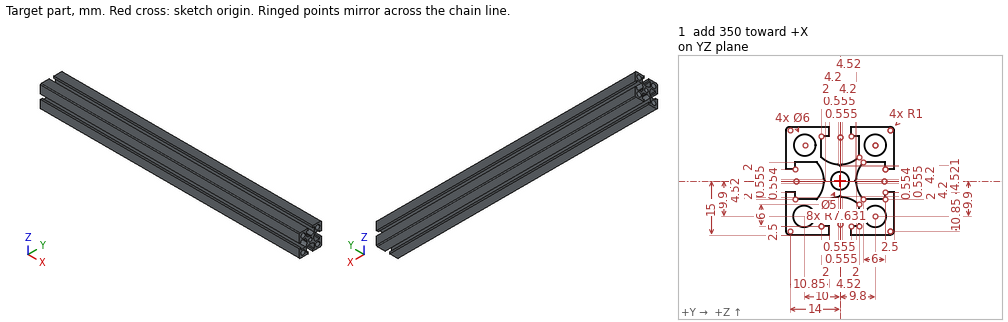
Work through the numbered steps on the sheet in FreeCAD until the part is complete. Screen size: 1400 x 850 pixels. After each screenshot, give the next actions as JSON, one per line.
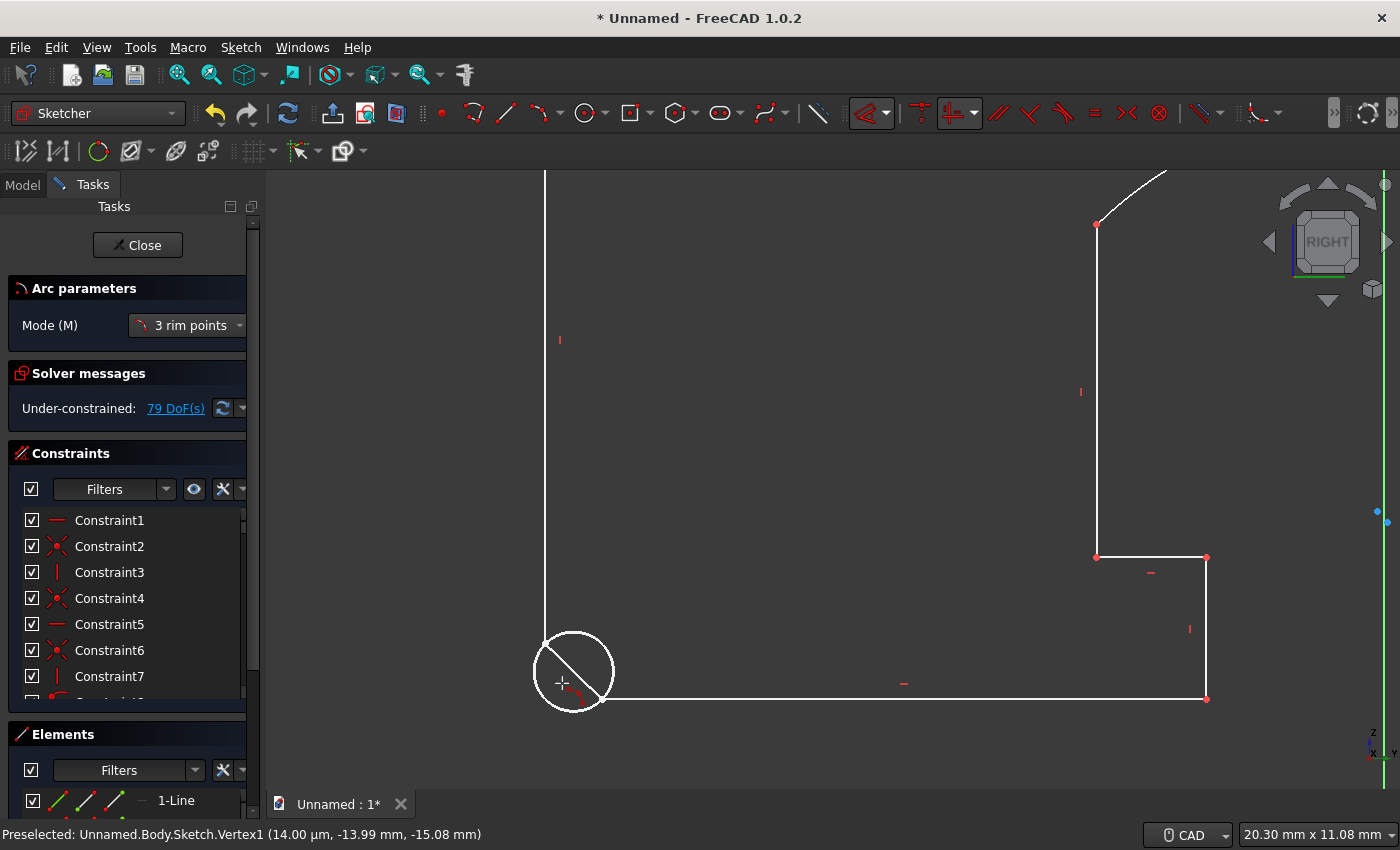
{"action": "left_click", "coordinate": [562, 679]}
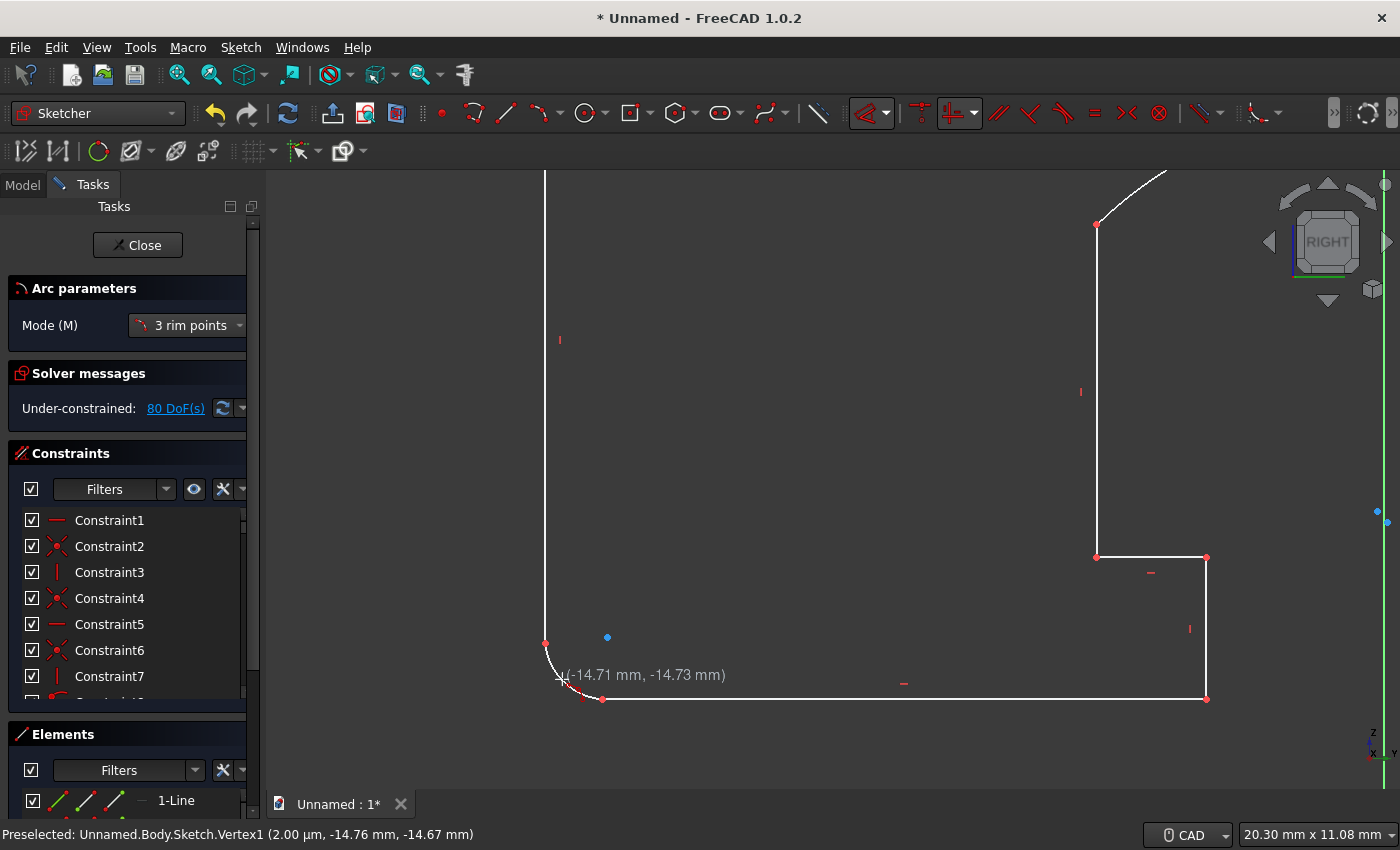
{"action": "left_click", "coordinate": [586, 114]}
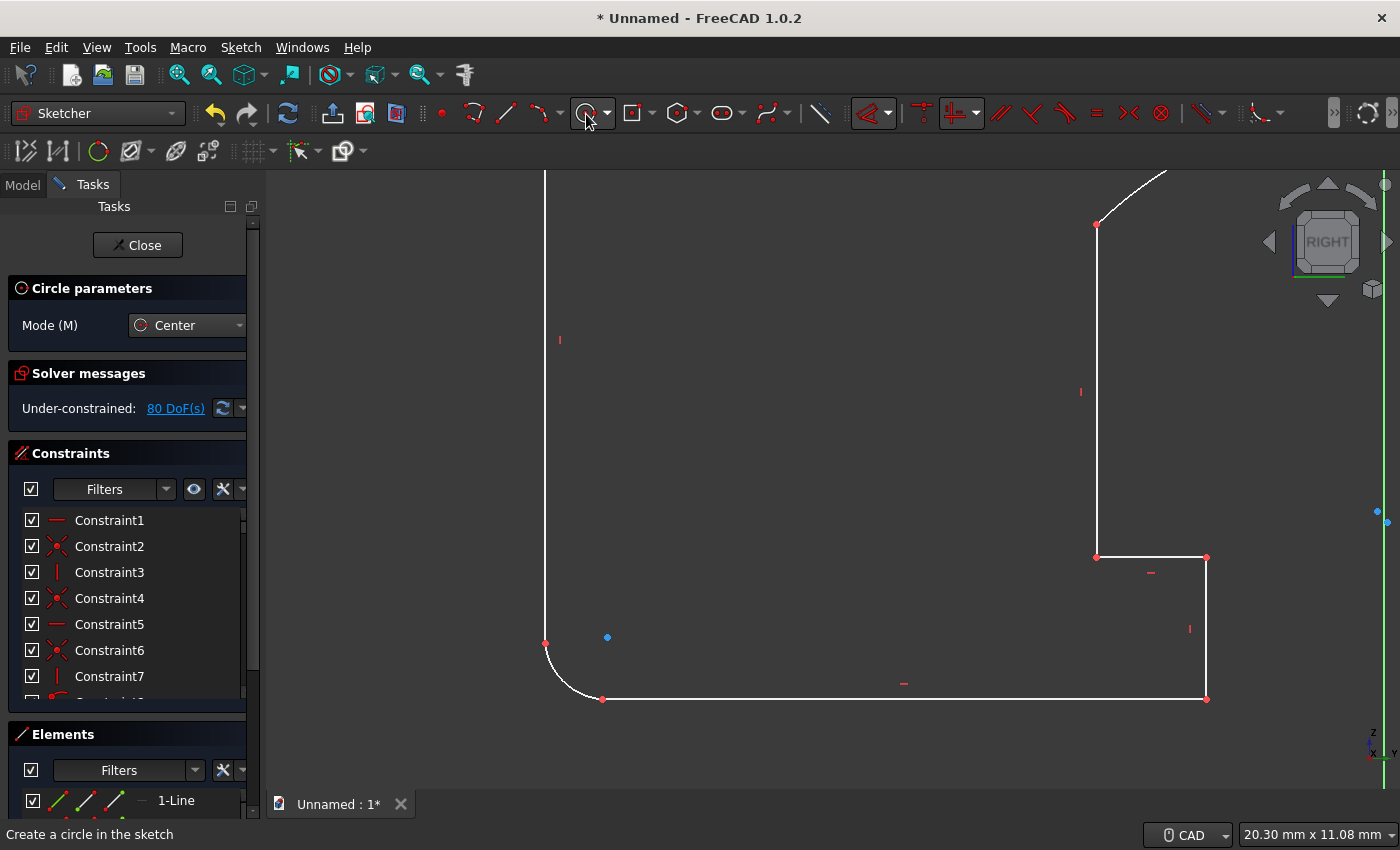
{"action": "scroll", "coordinate": [562, 683], "scroll_direction": "down", "scroll_amount": 7}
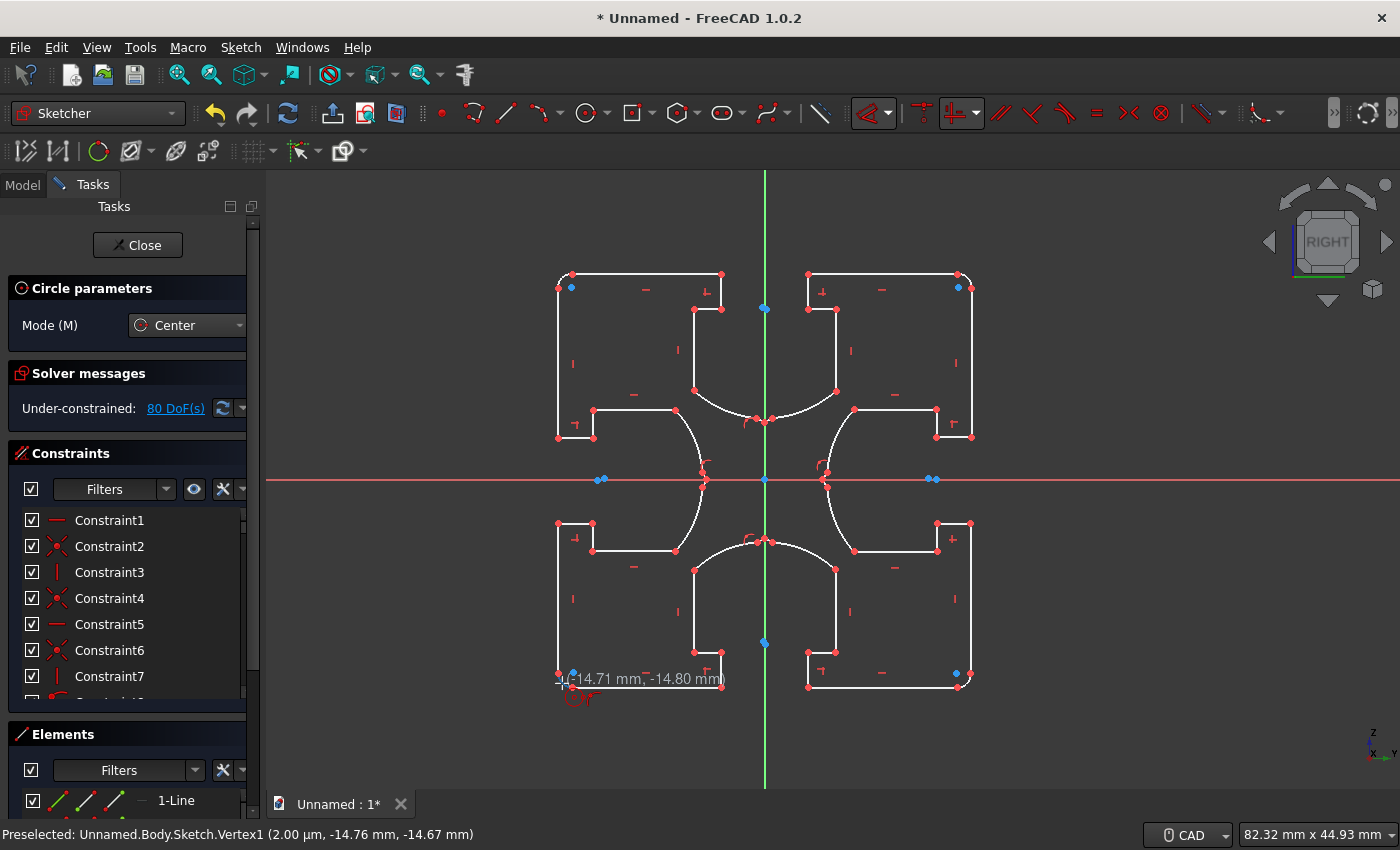
{"action": "left_click", "coordinate": [627, 616]}
{"action": "left_click", "coordinate": [656, 587]}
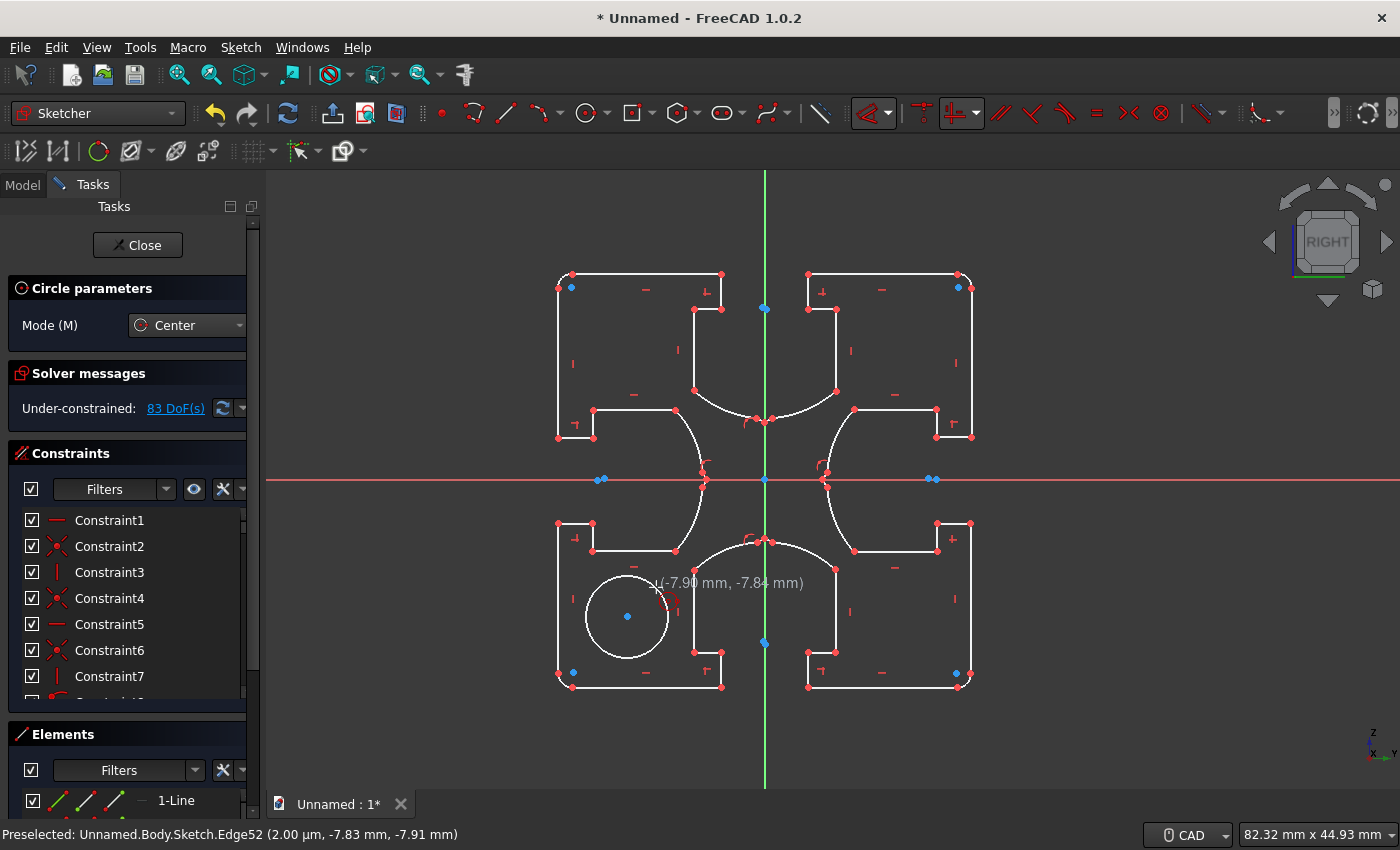
{"action": "left_click", "coordinate": [900, 616]}
{"action": "left_click", "coordinate": [929, 587]}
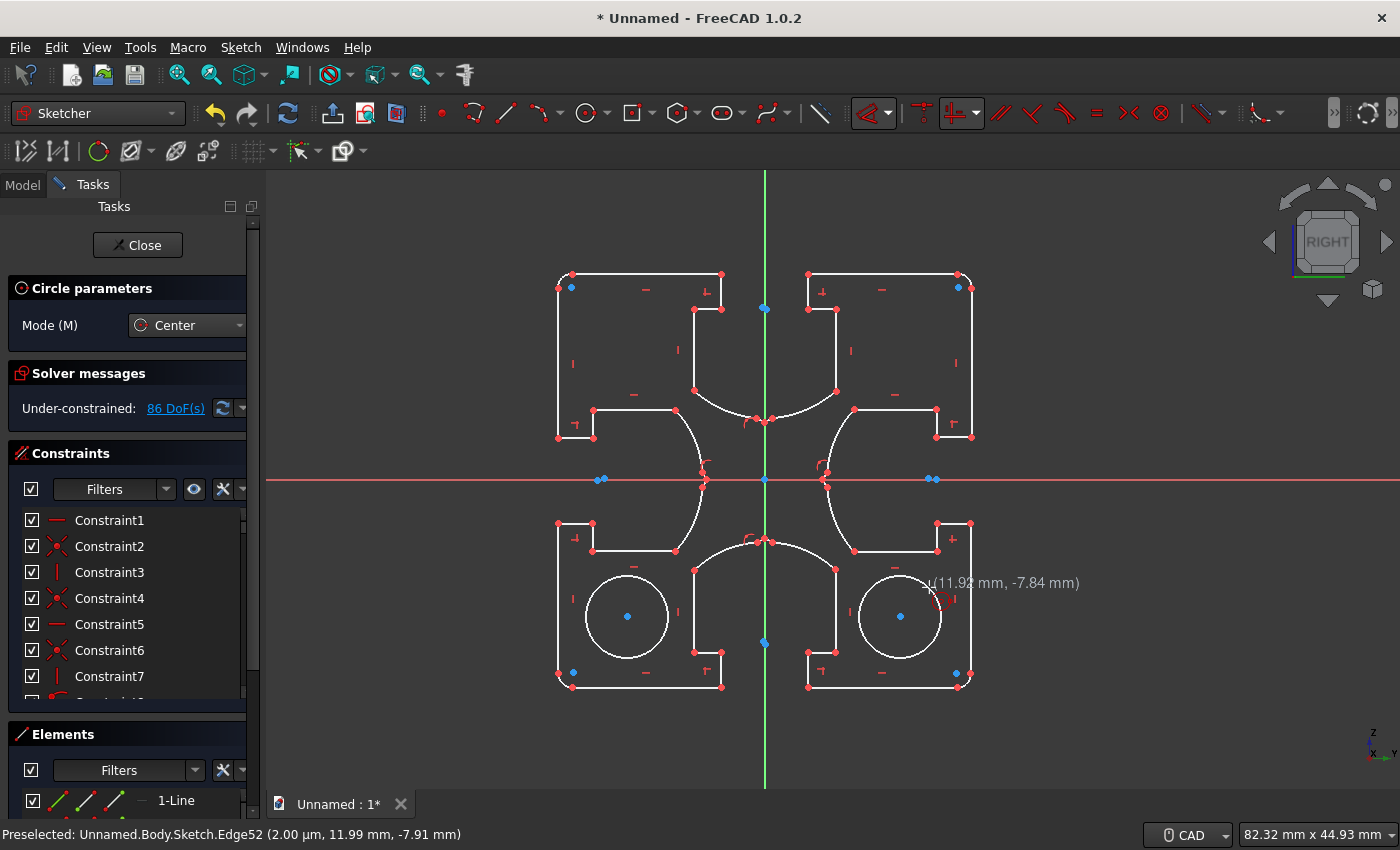
{"action": "left_click", "coordinate": [630, 344]}
{"action": "left_click", "coordinate": [659, 314]}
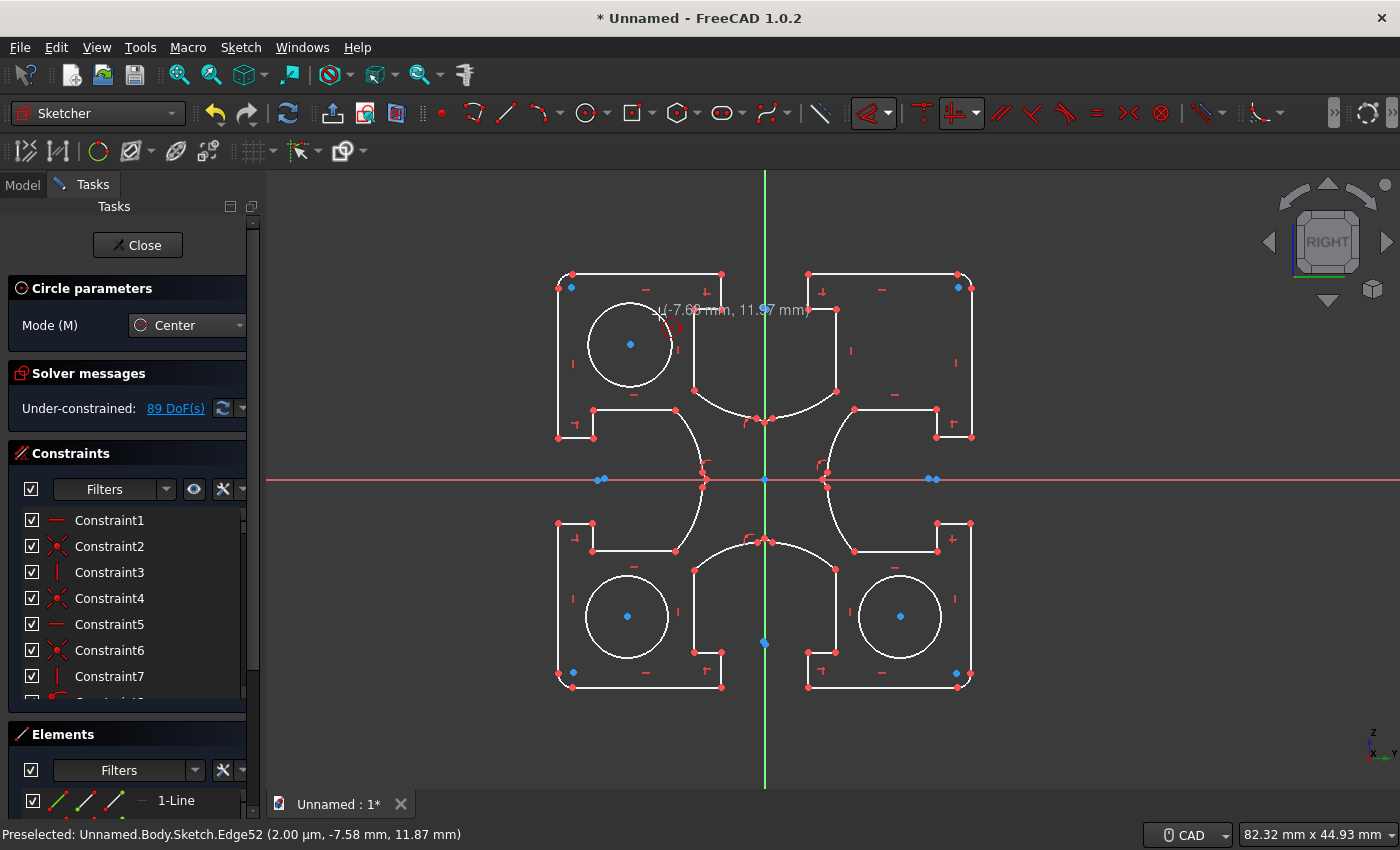
{"action": "left_click", "coordinate": [765, 480]}
{"action": "left_click", "coordinate": [789, 456]}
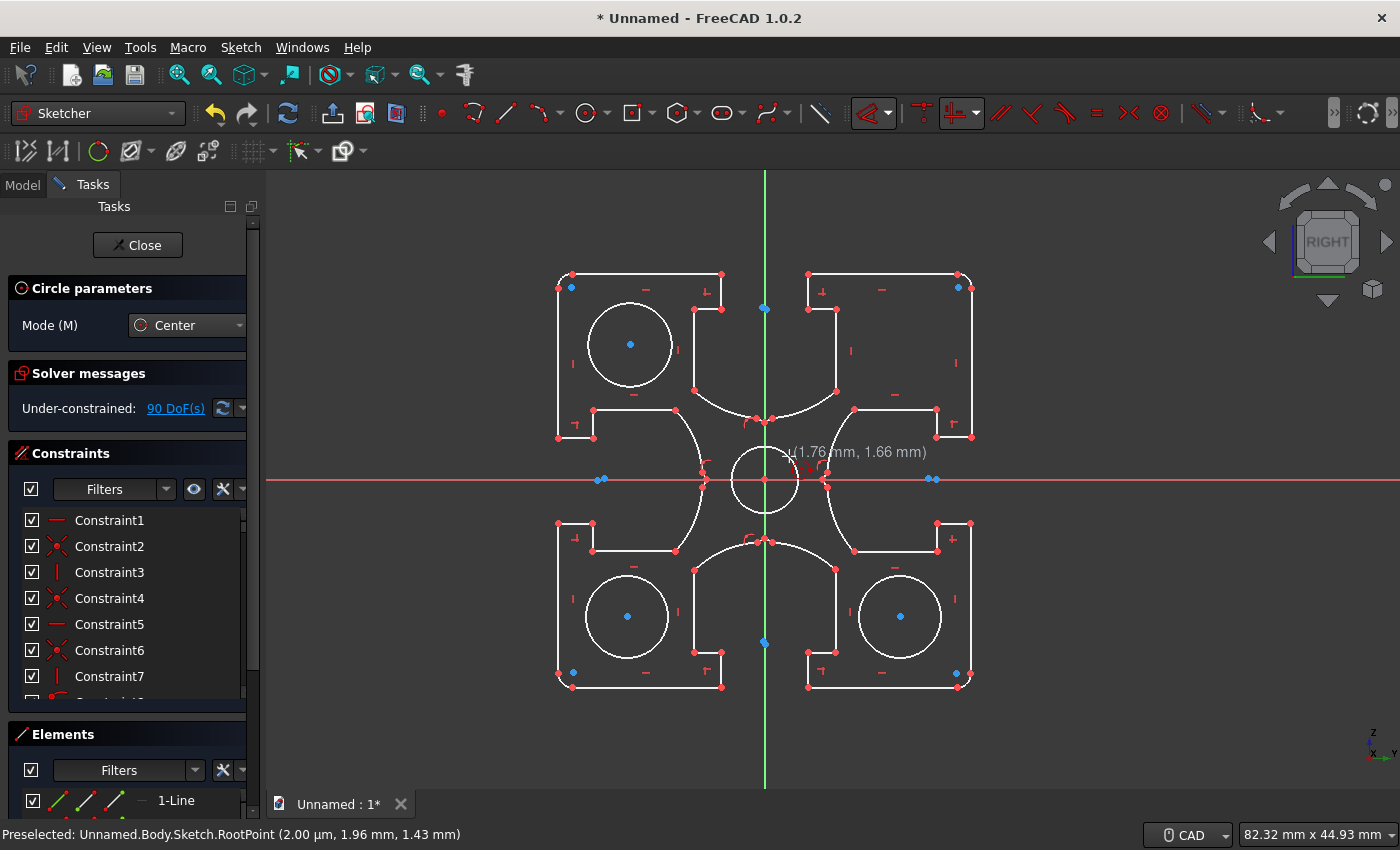
{"action": "left_click", "coordinate": [900, 344]}
{"action": "left_click", "coordinate": [929, 314]}
{"action": "key", "text": "Escape"}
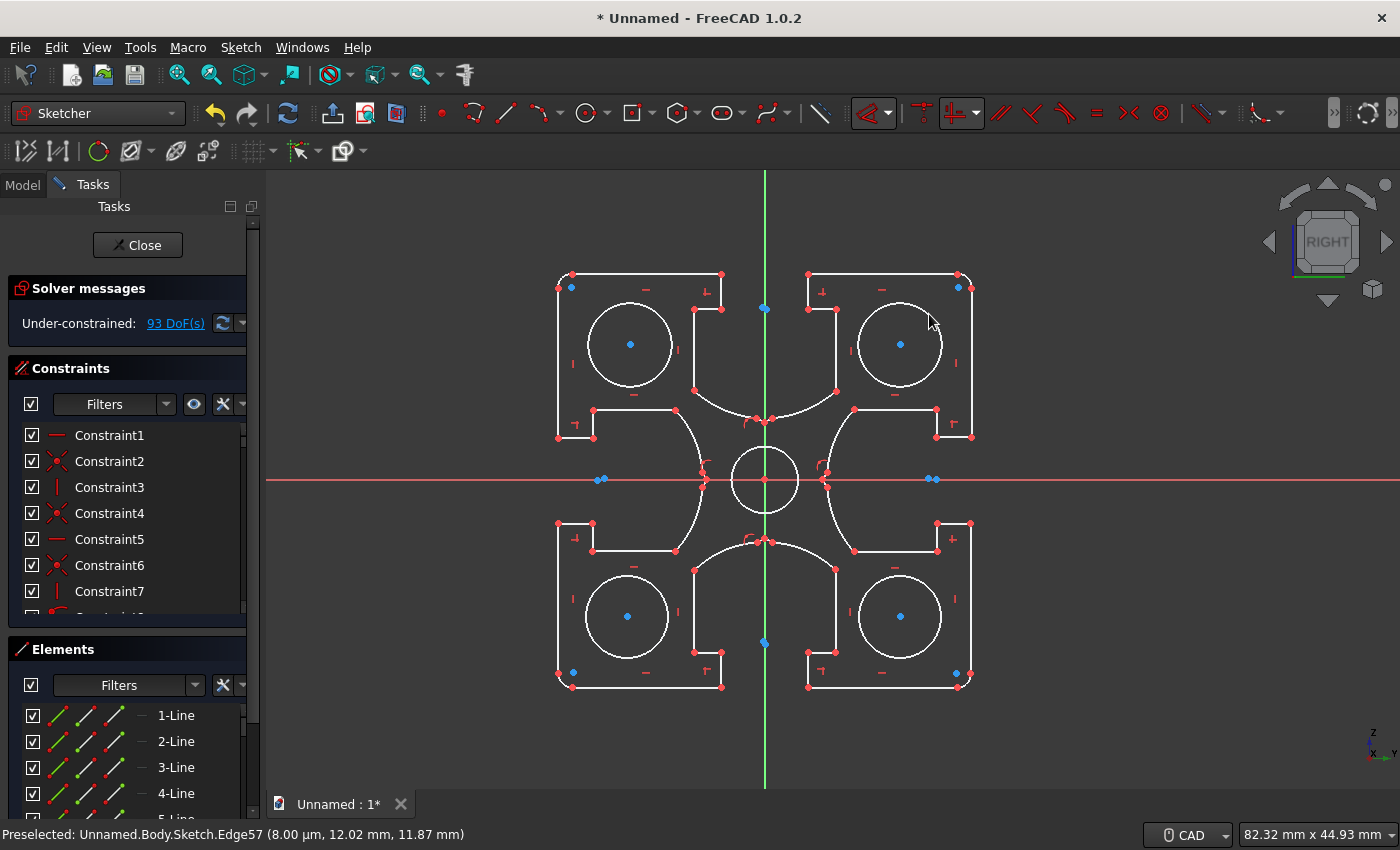
{"action": "left_click", "coordinate": [617, 688]}